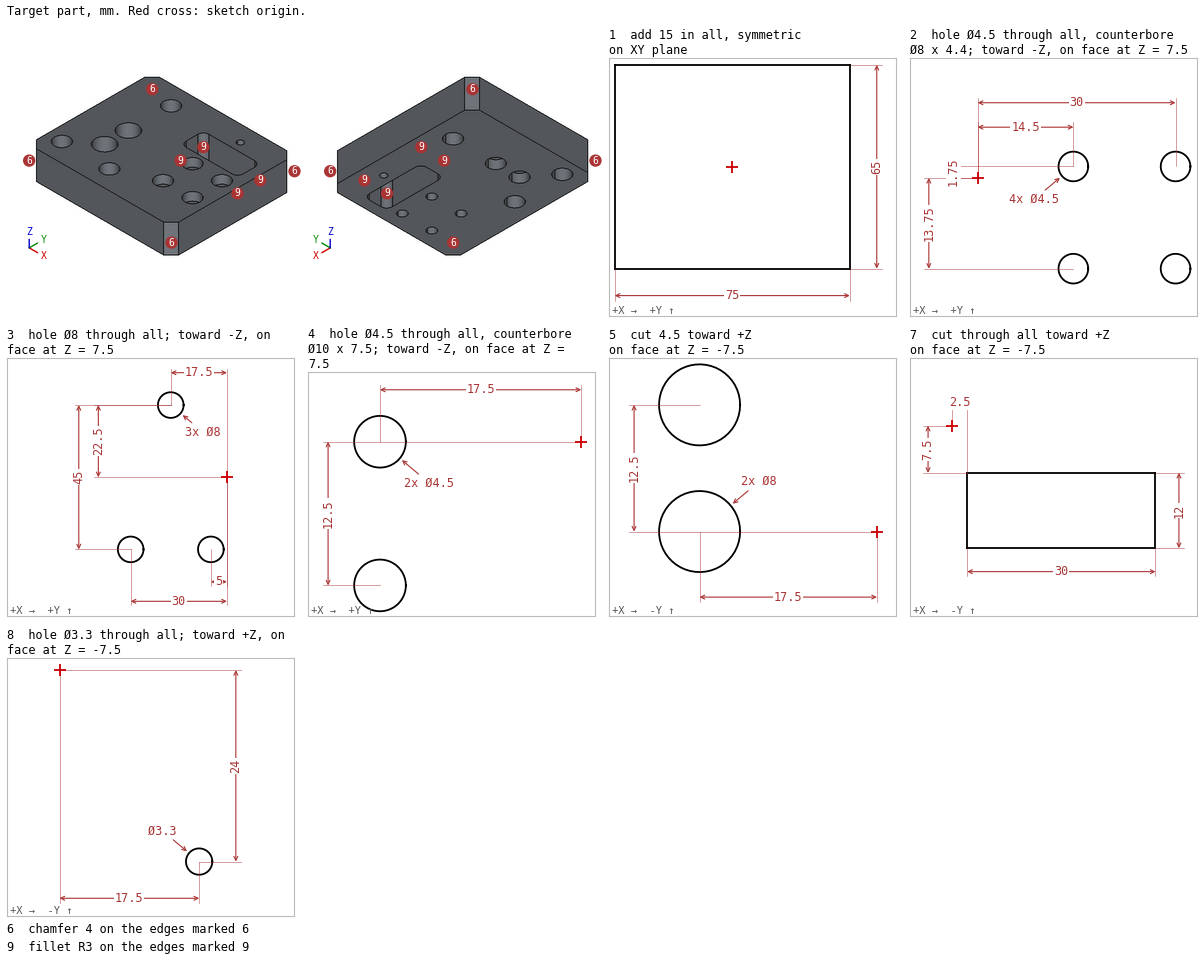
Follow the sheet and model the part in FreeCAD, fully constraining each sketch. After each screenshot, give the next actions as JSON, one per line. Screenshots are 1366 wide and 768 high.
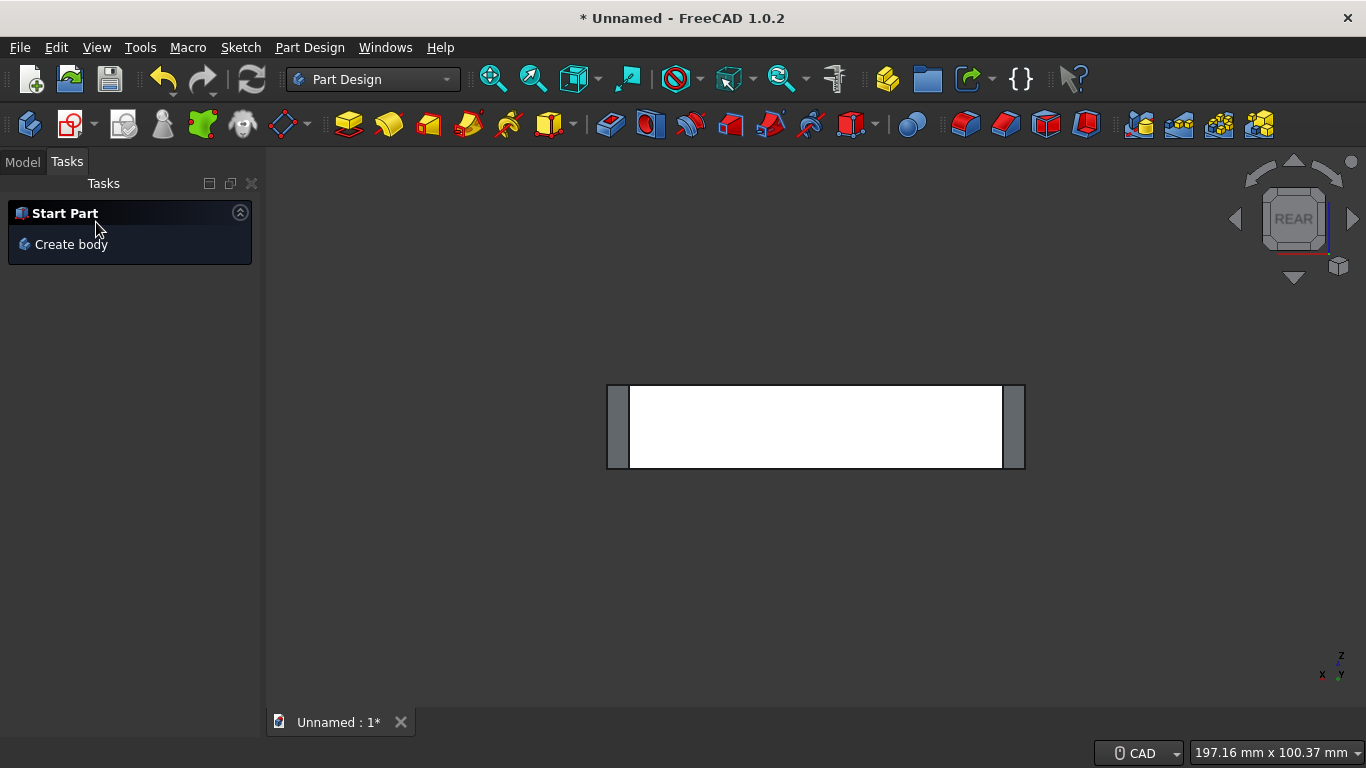
{"action": "key", "text": "v f"}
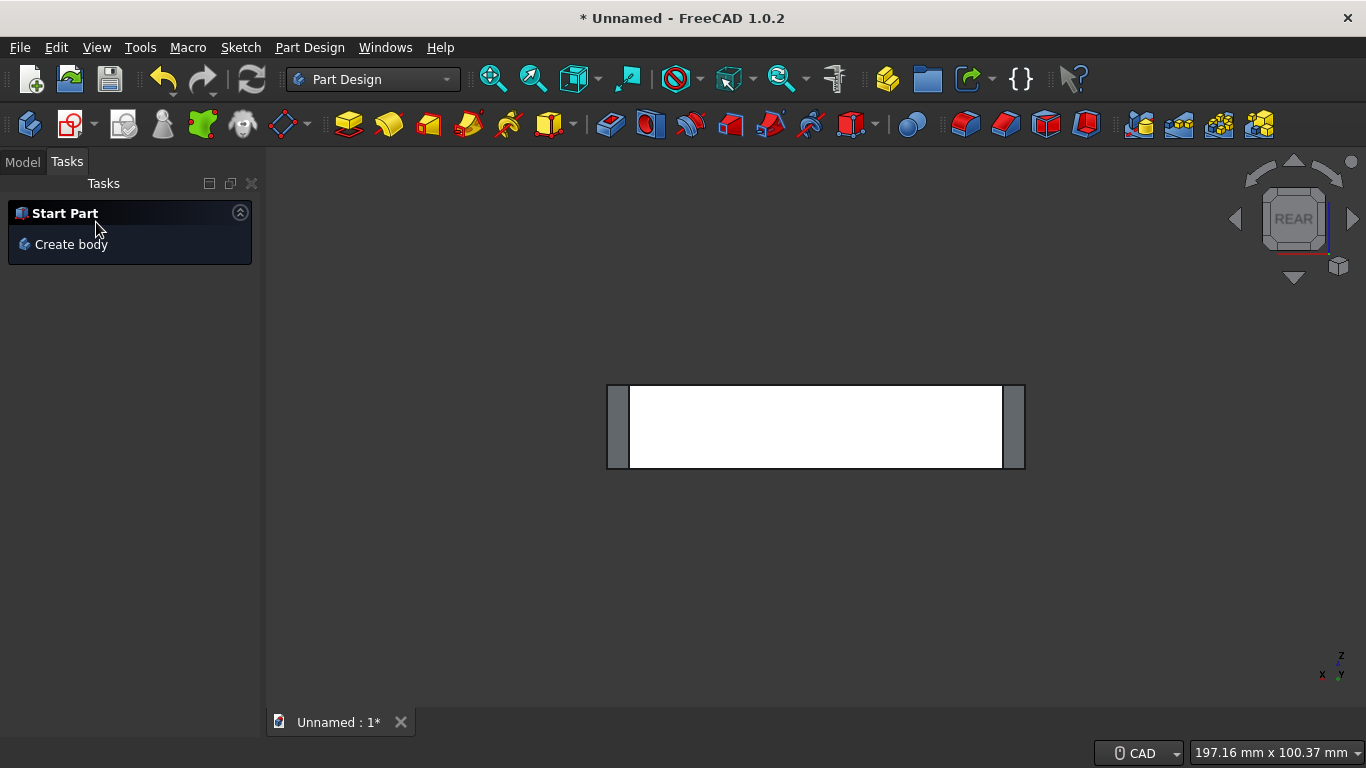
{"action": "key", "text": "5"}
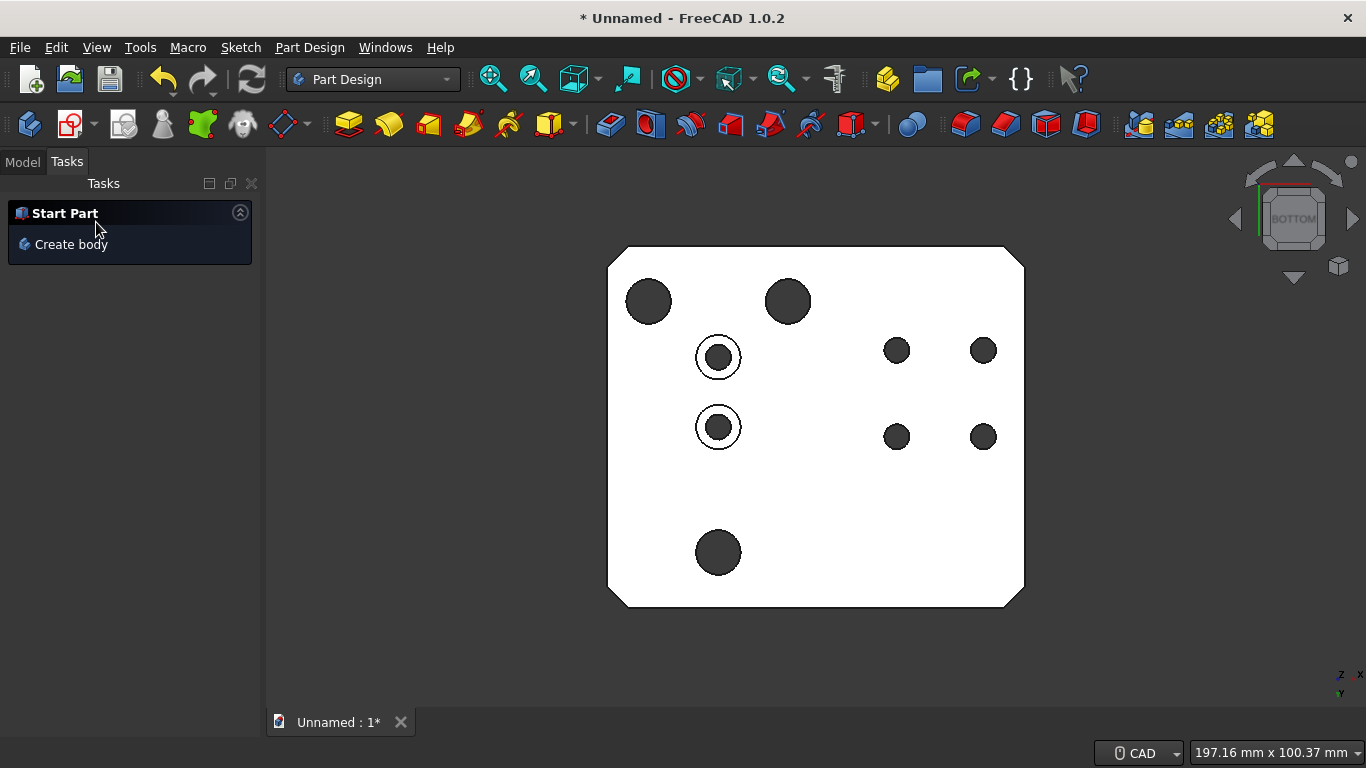
{"action": "left_click", "coordinate": [816, 478]}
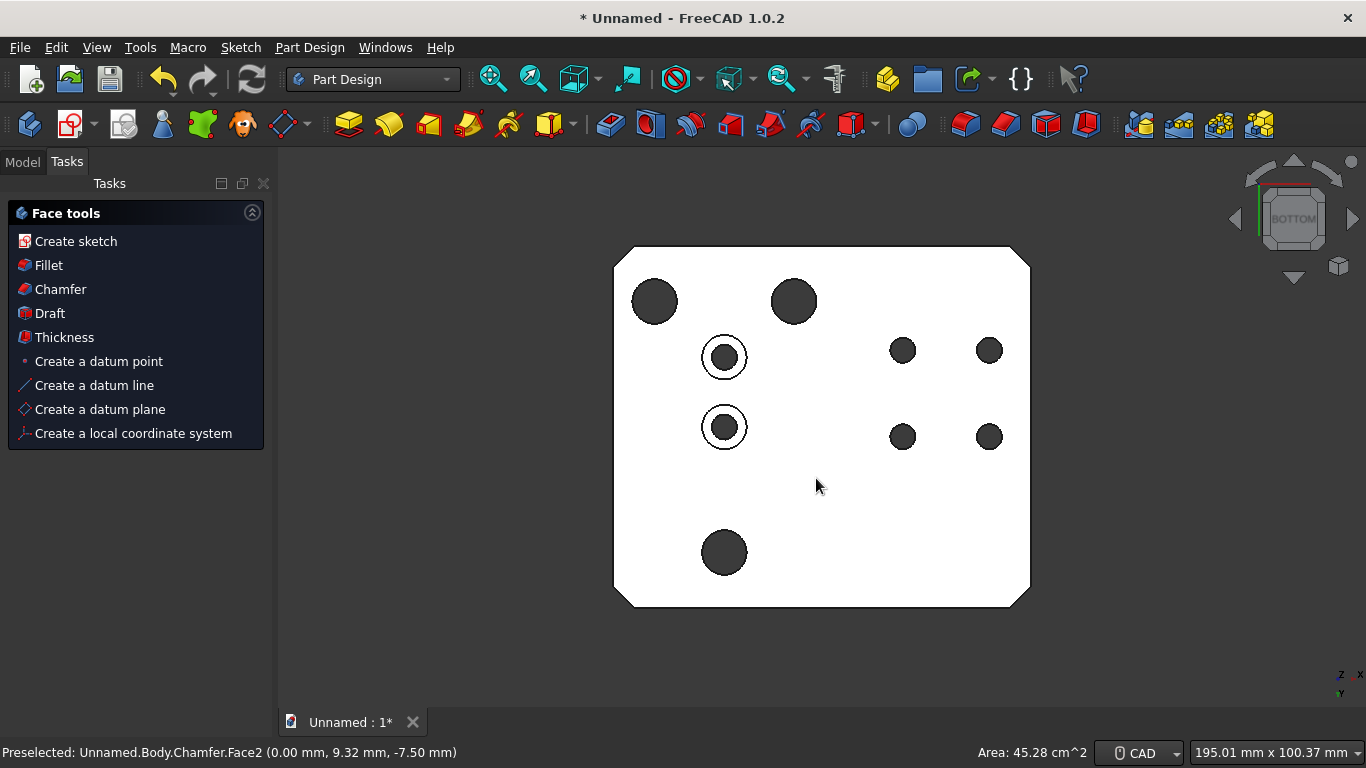
{"action": "left_click", "coordinate": [70, 124]}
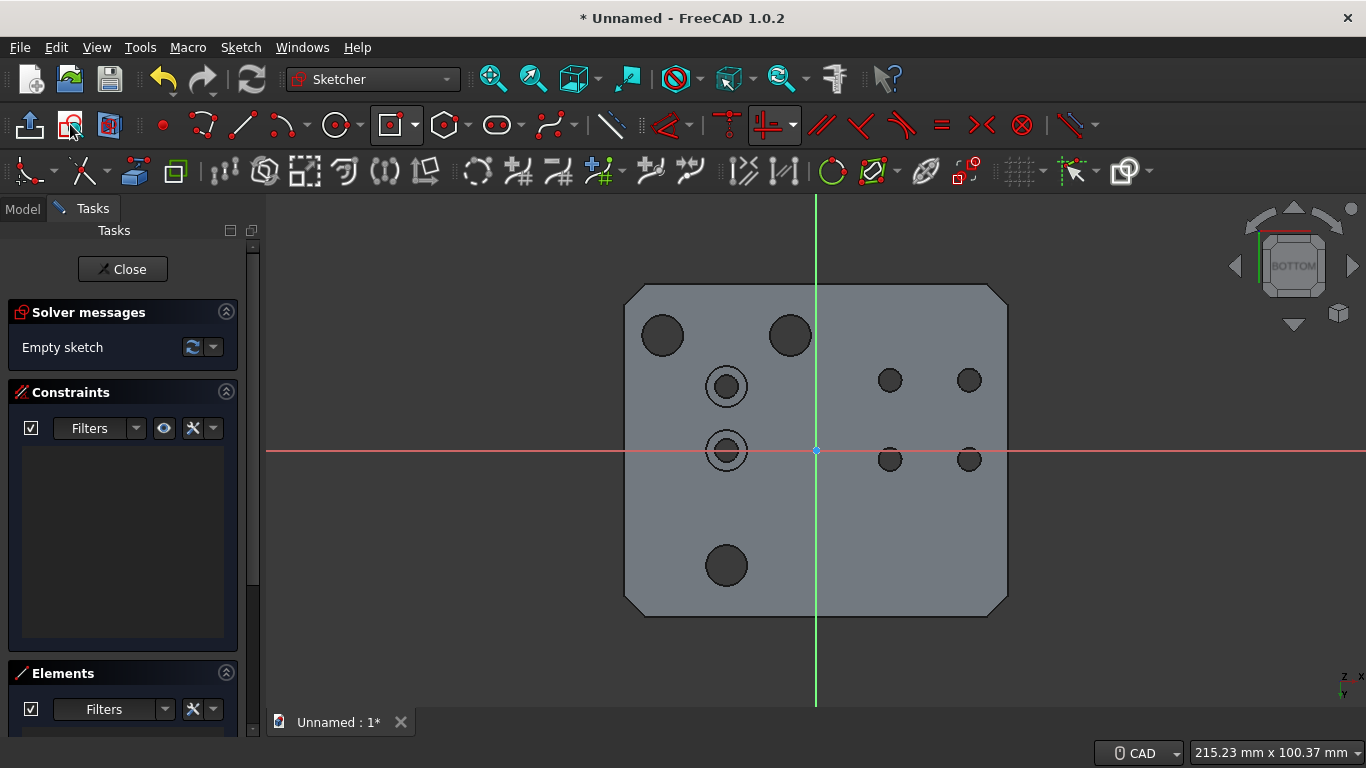
{"action": "scroll", "coordinate": [964, 522], "scroll_direction": "up", "scroll_amount": 6}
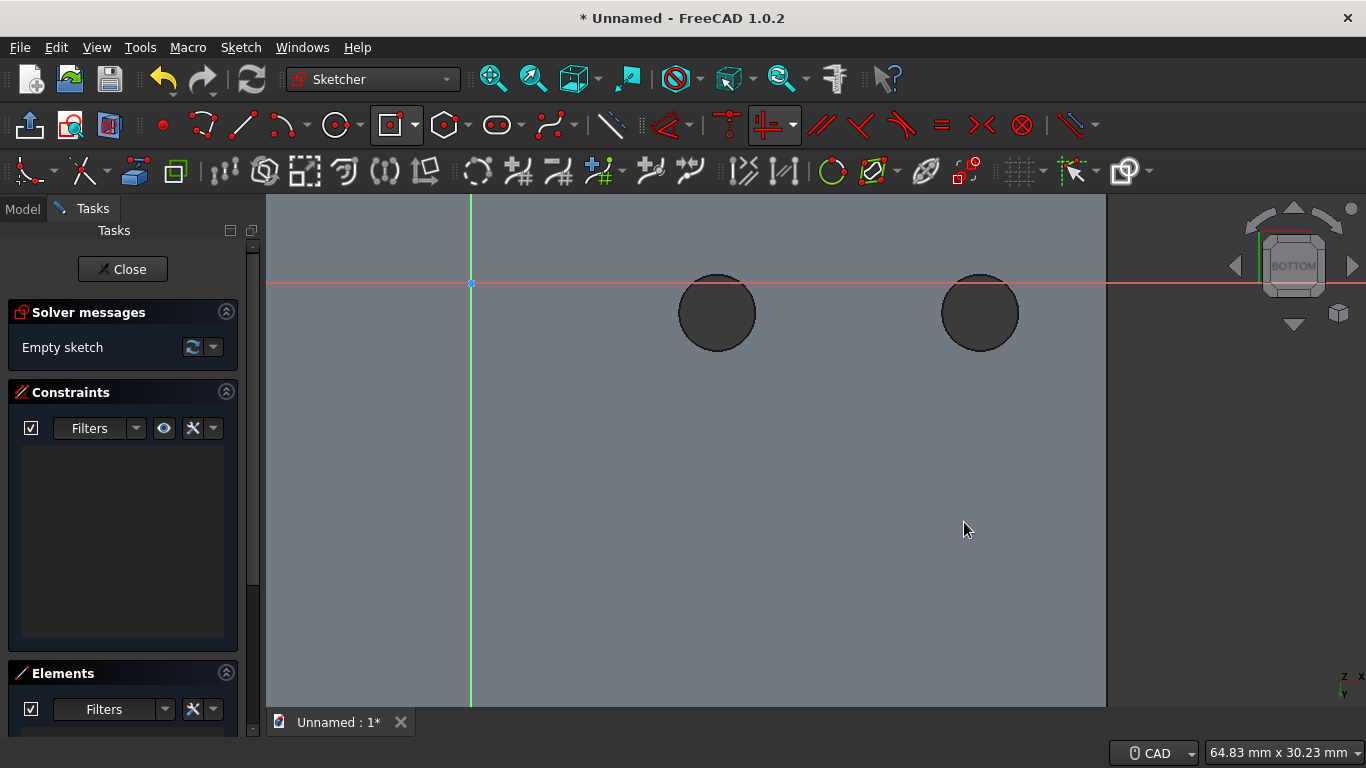
{"action": "key", "text": "g r"}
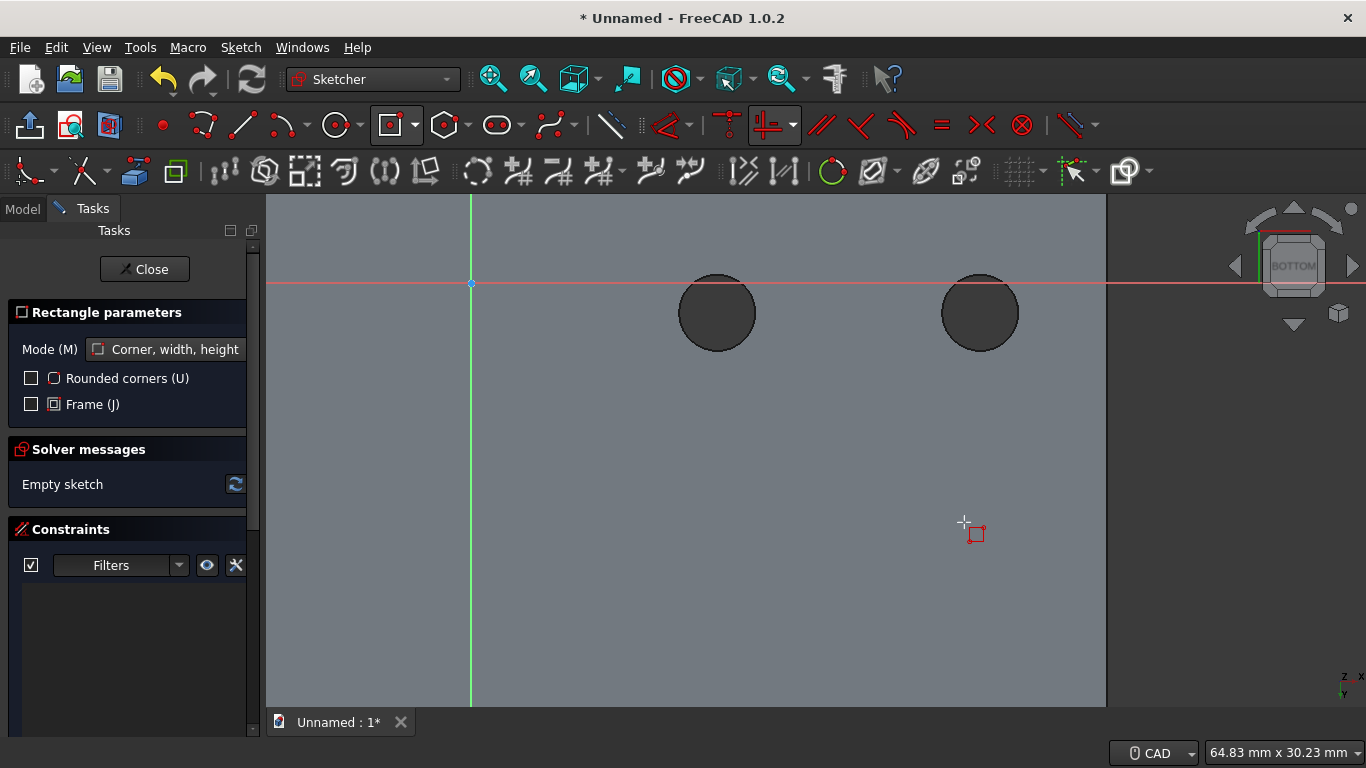
{"action": "left_click", "coordinate": [514, 410]}
{"action": "mouse_move", "coordinate": [1023, 614]}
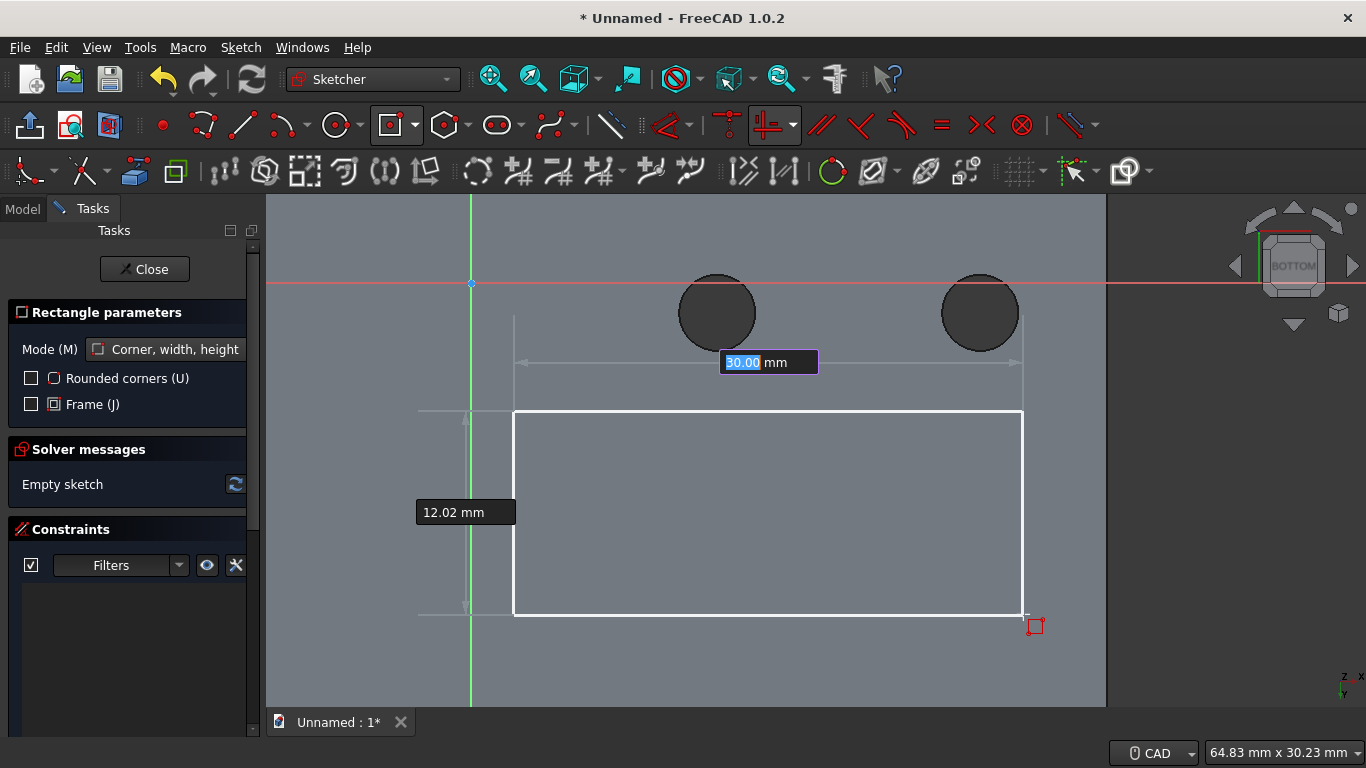
{"action": "type", "text": "30"}
{"action": "key", "text": "Tab"}
{"action": "type", "text": "12"}
{"action": "key", "text": "Return"}
{"action": "key", "text": "Escape"}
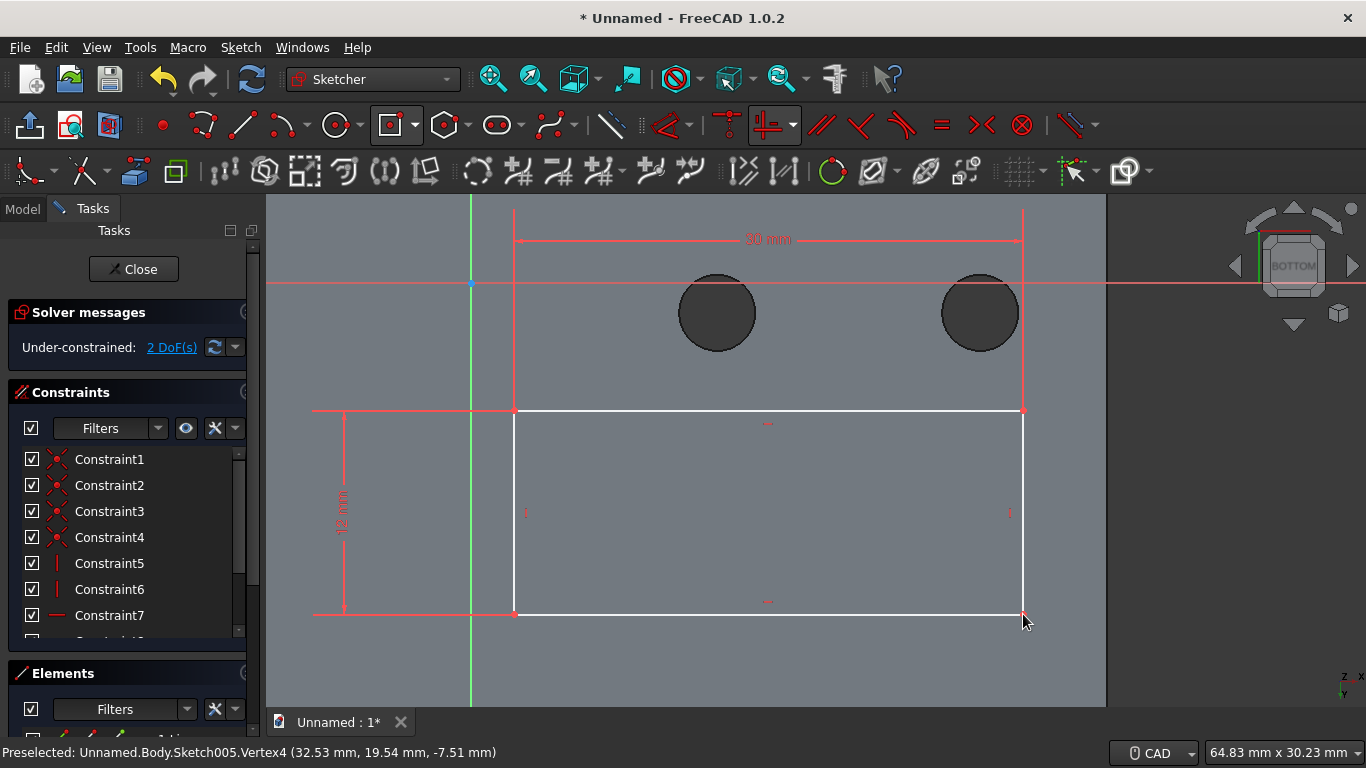
{"action": "left_click", "coordinate": [514, 411]}